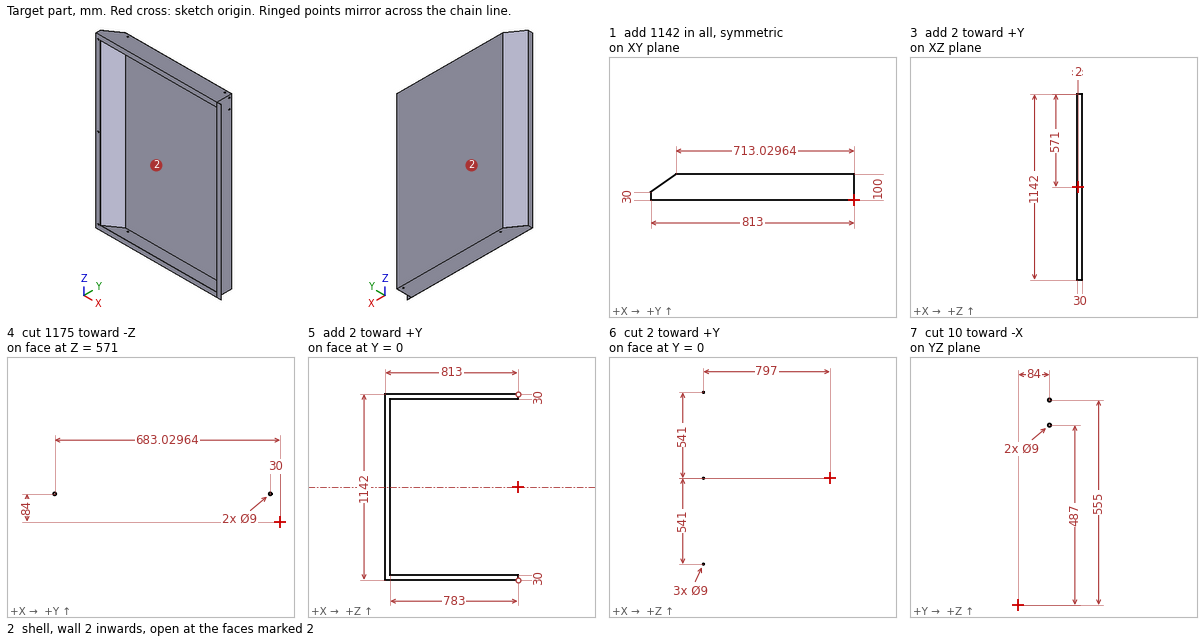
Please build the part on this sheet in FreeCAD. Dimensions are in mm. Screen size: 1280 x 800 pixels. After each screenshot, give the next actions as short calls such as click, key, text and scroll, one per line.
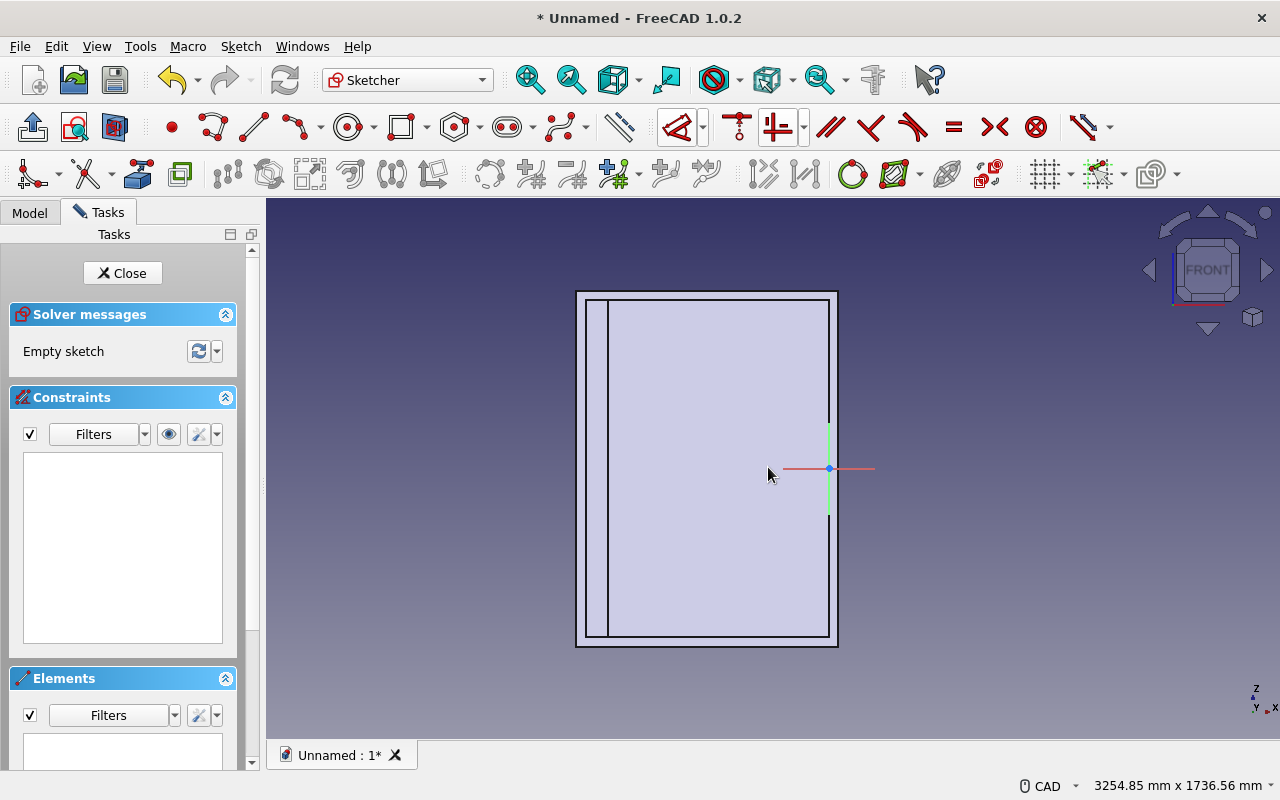
click(348, 128)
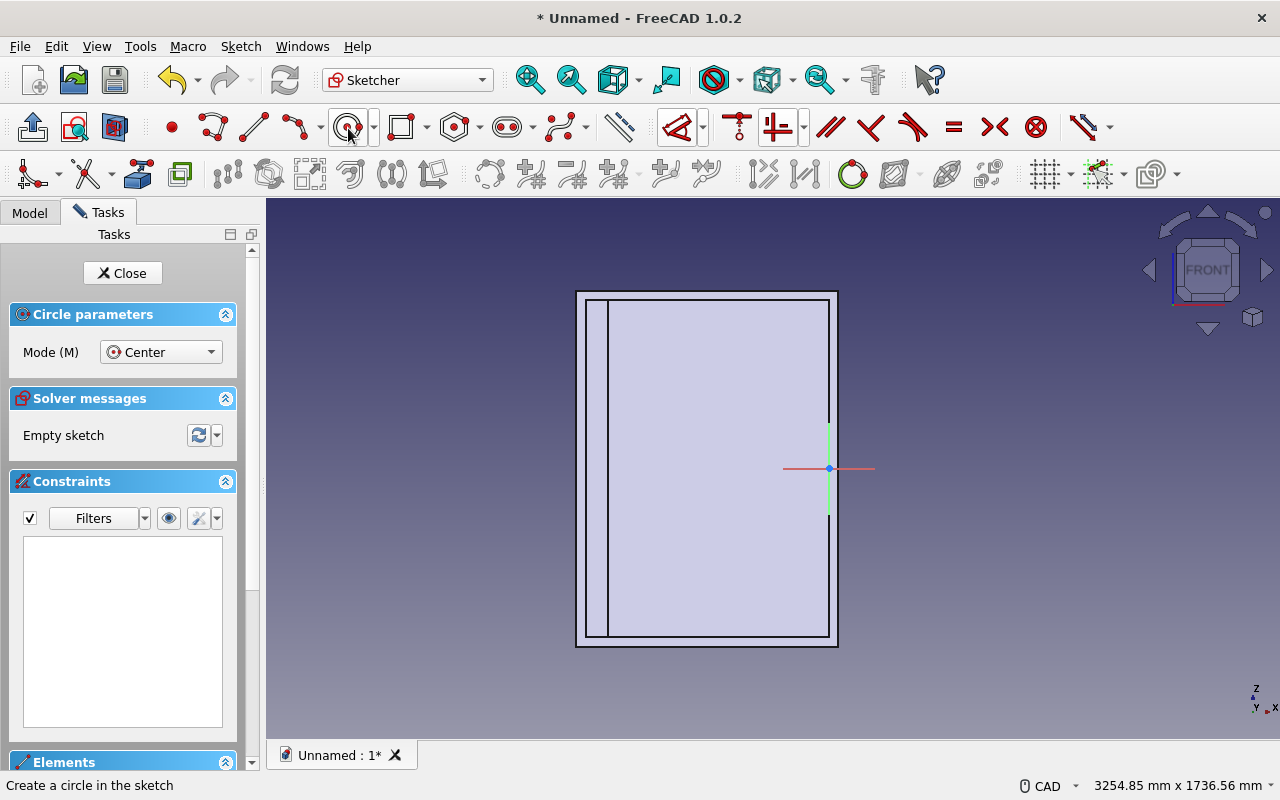
scroll(581, 300, up, 14)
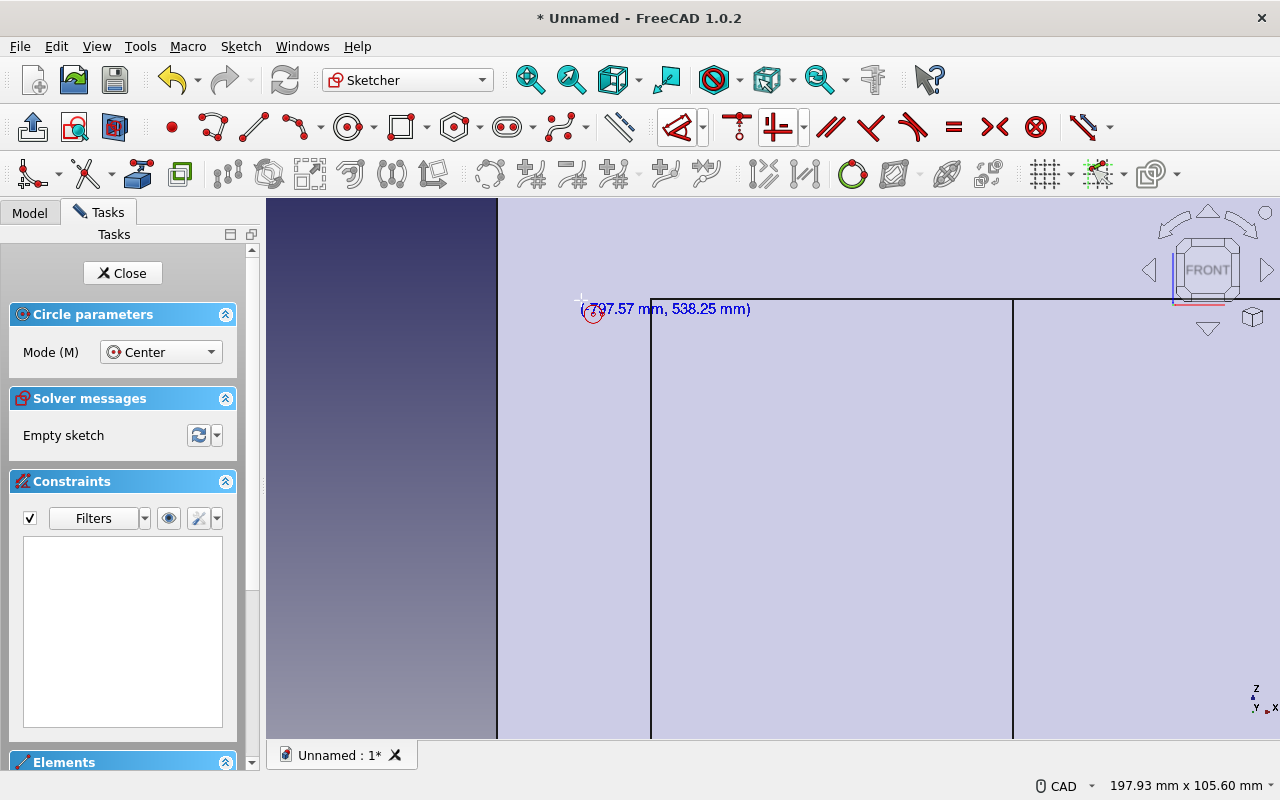
scroll(581, 300, down, 14)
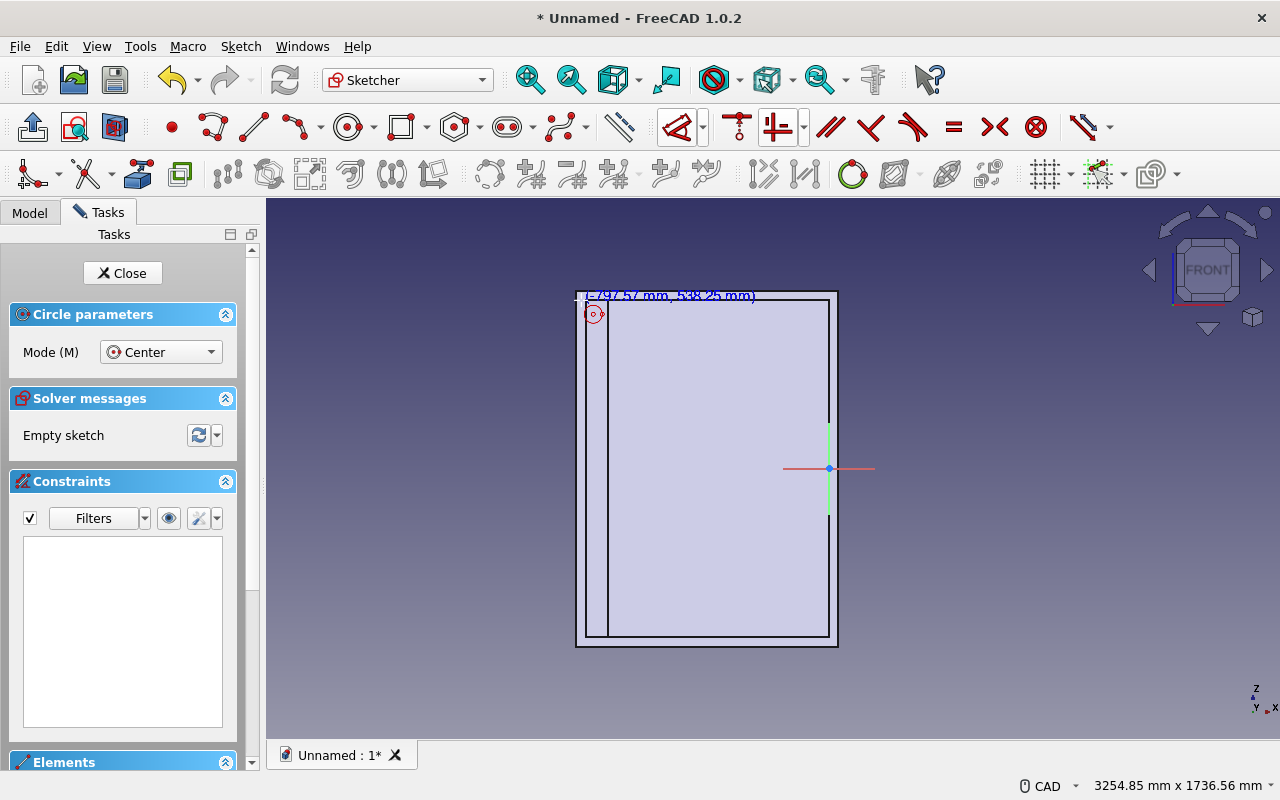
click(581, 300)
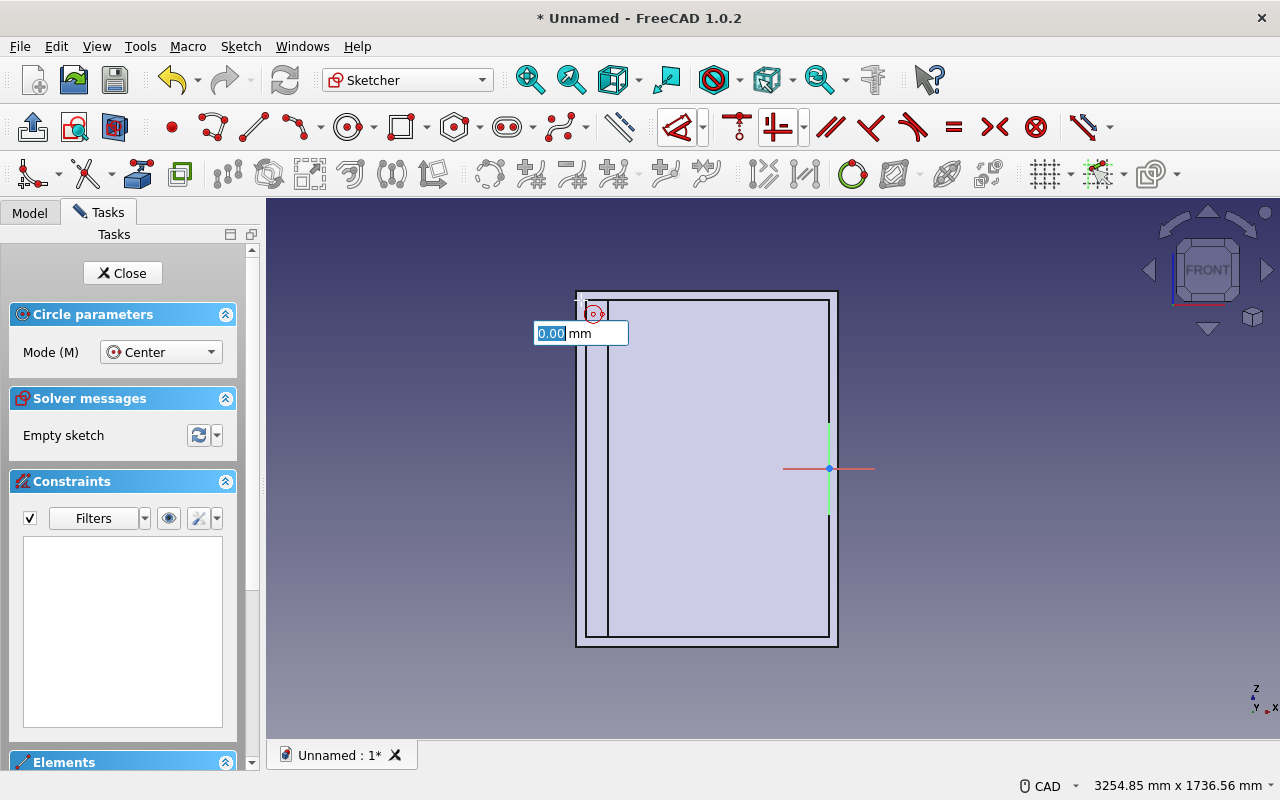
scroll(582, 299, up, 13)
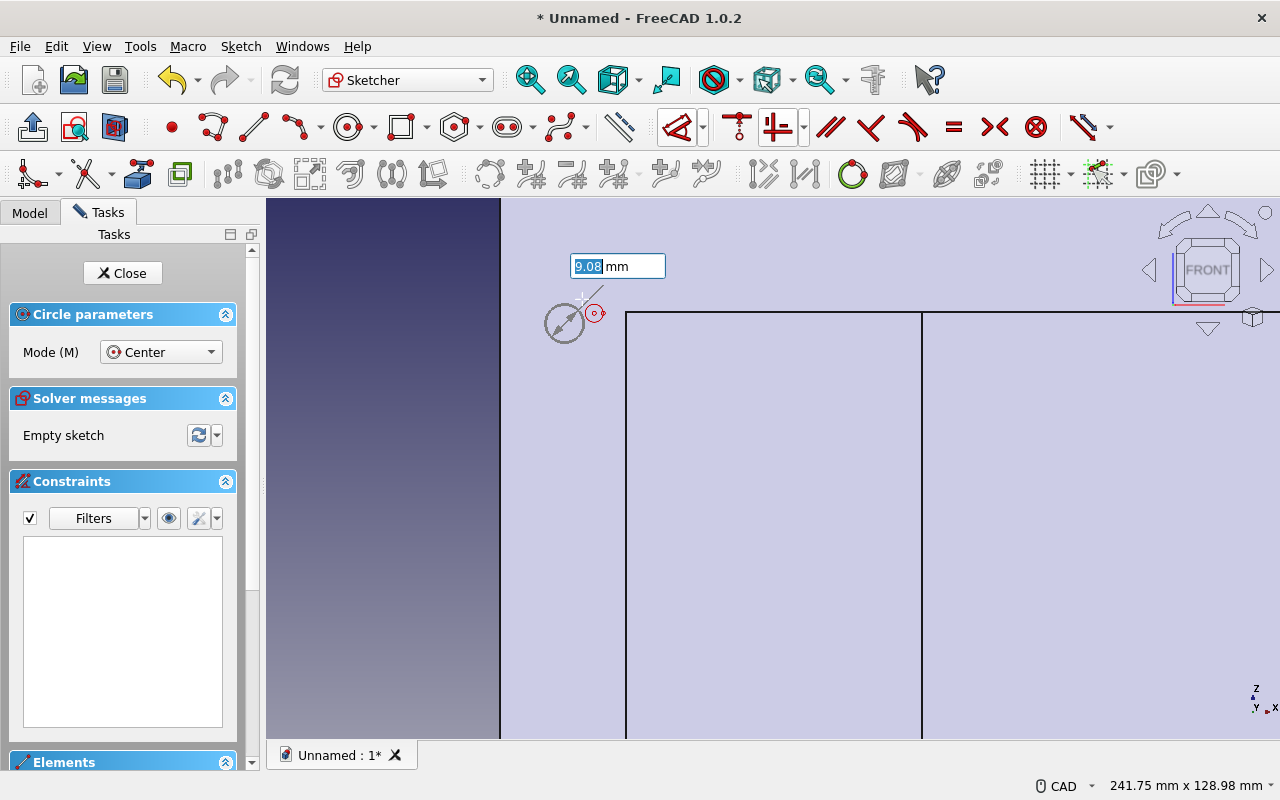
click(580, 299)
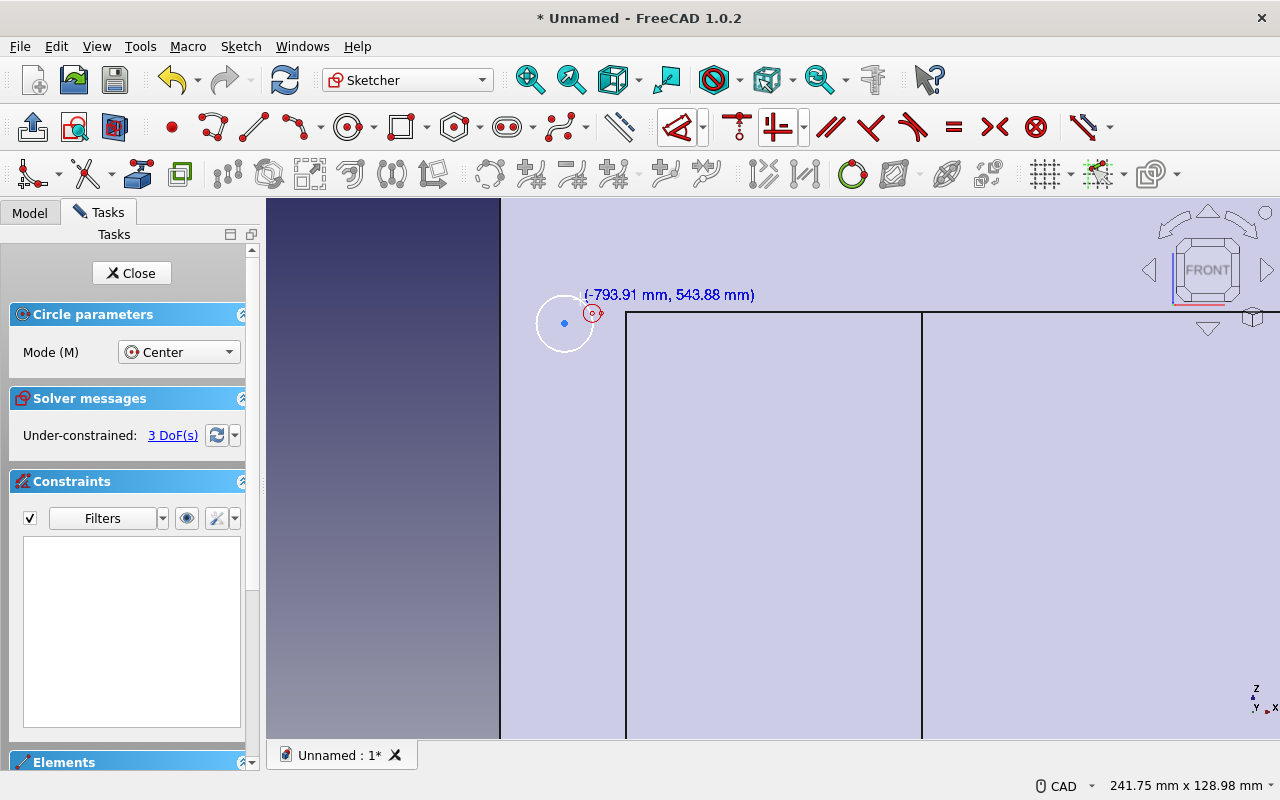
scroll(582, 299, down, 13)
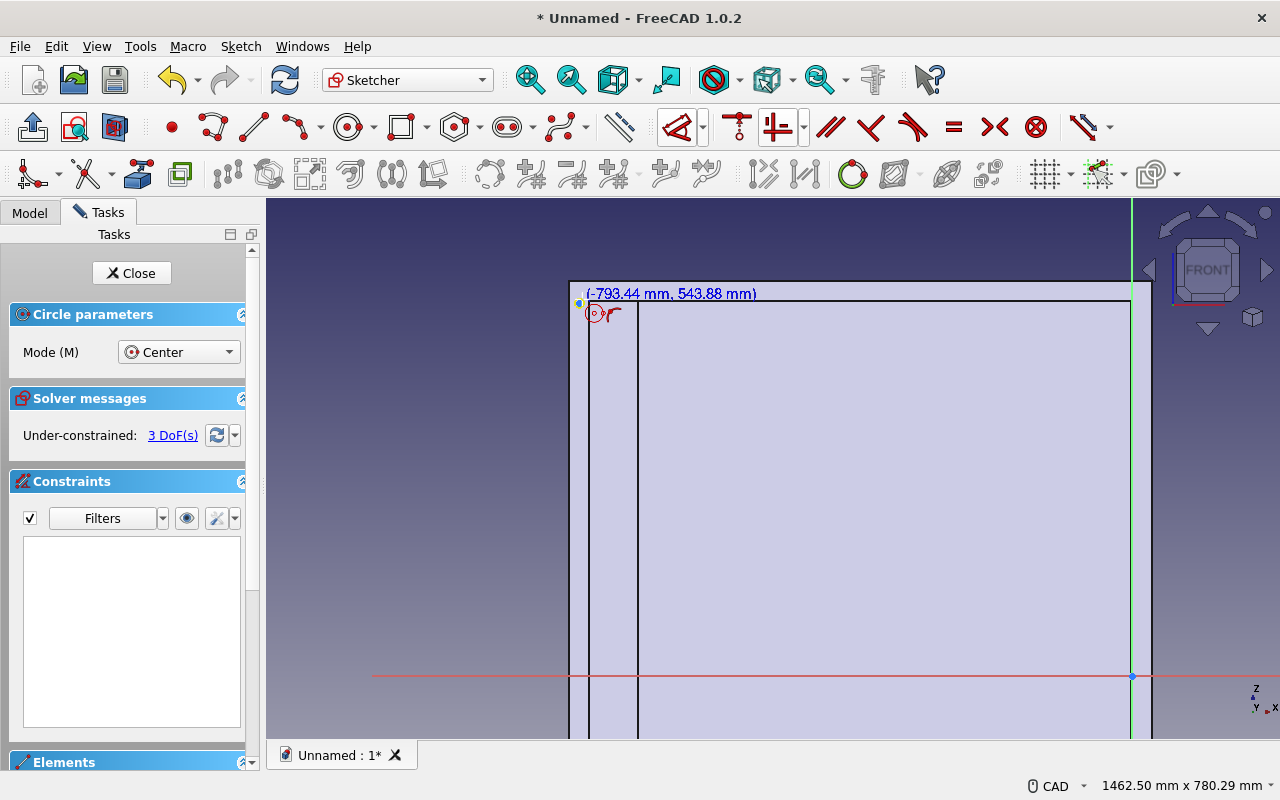
scroll(581, 637, up, 14)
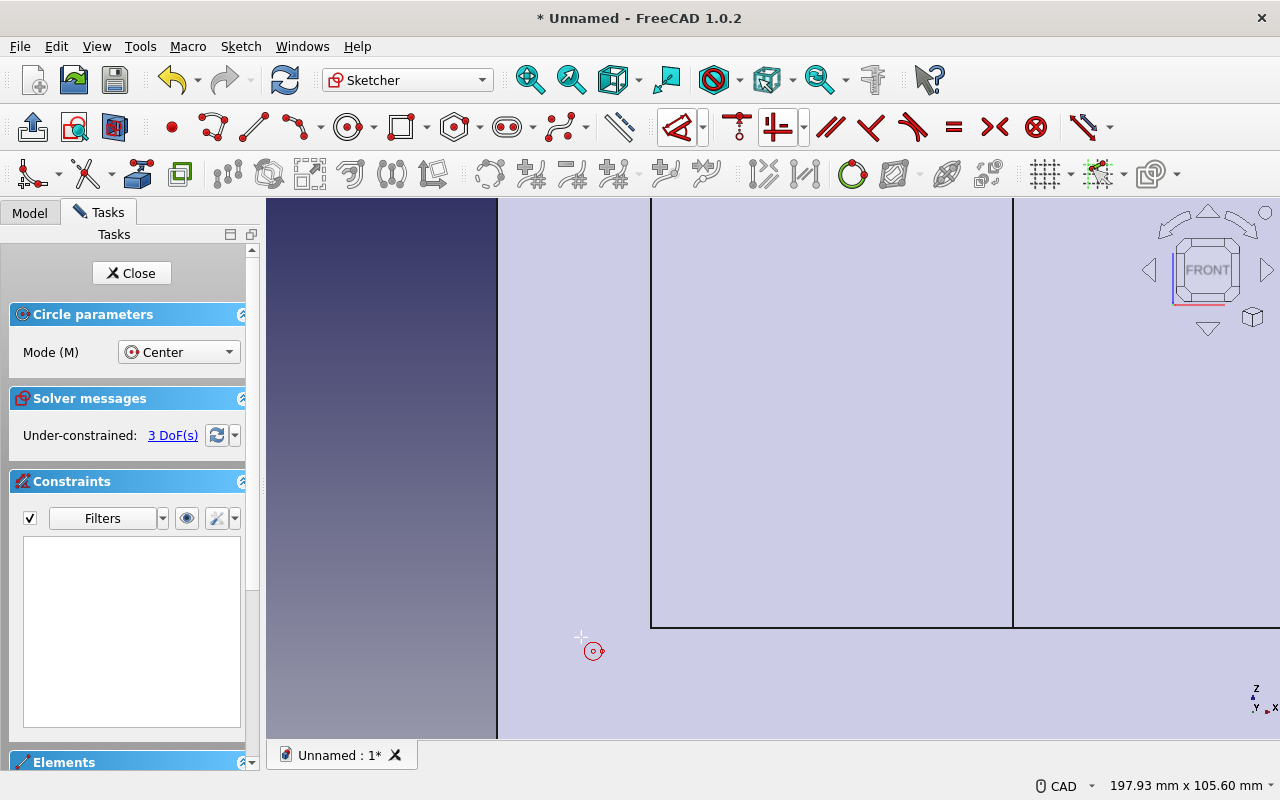
scroll(581, 638, down, 14)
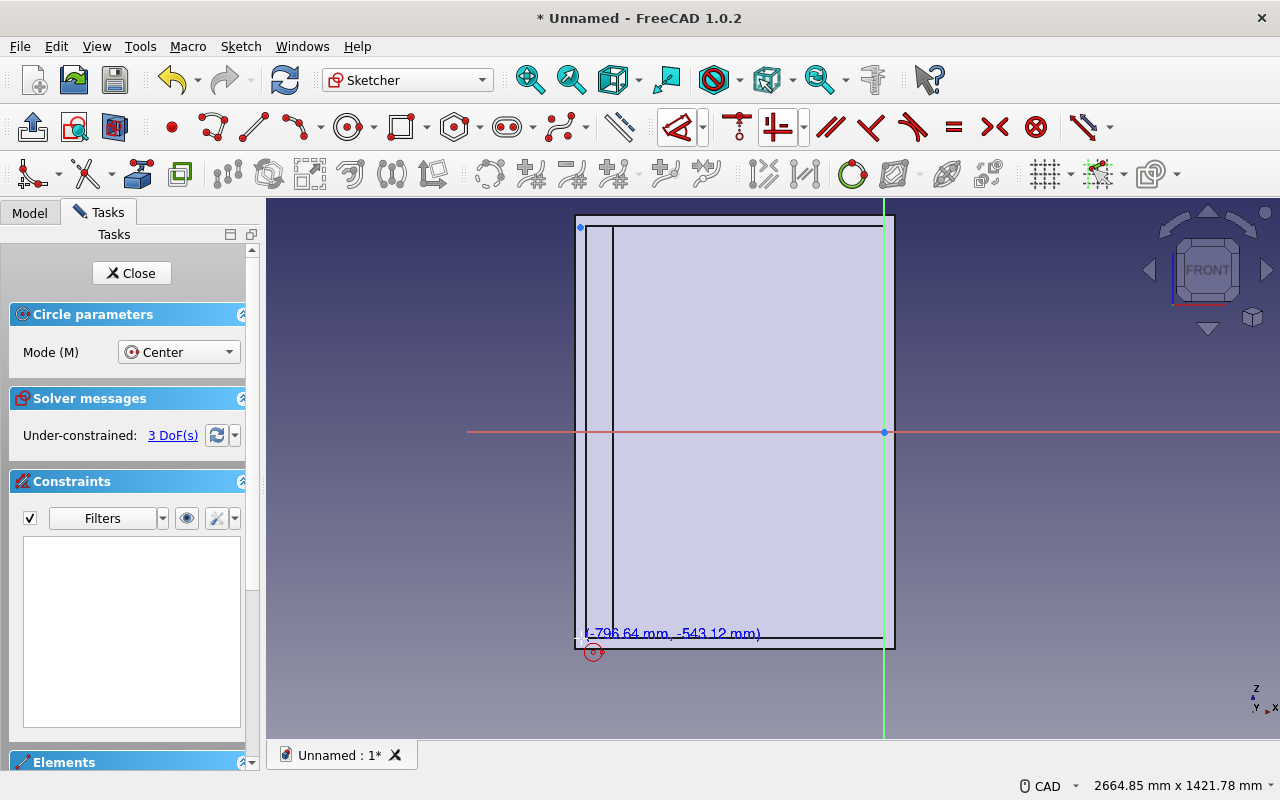
click(581, 638)